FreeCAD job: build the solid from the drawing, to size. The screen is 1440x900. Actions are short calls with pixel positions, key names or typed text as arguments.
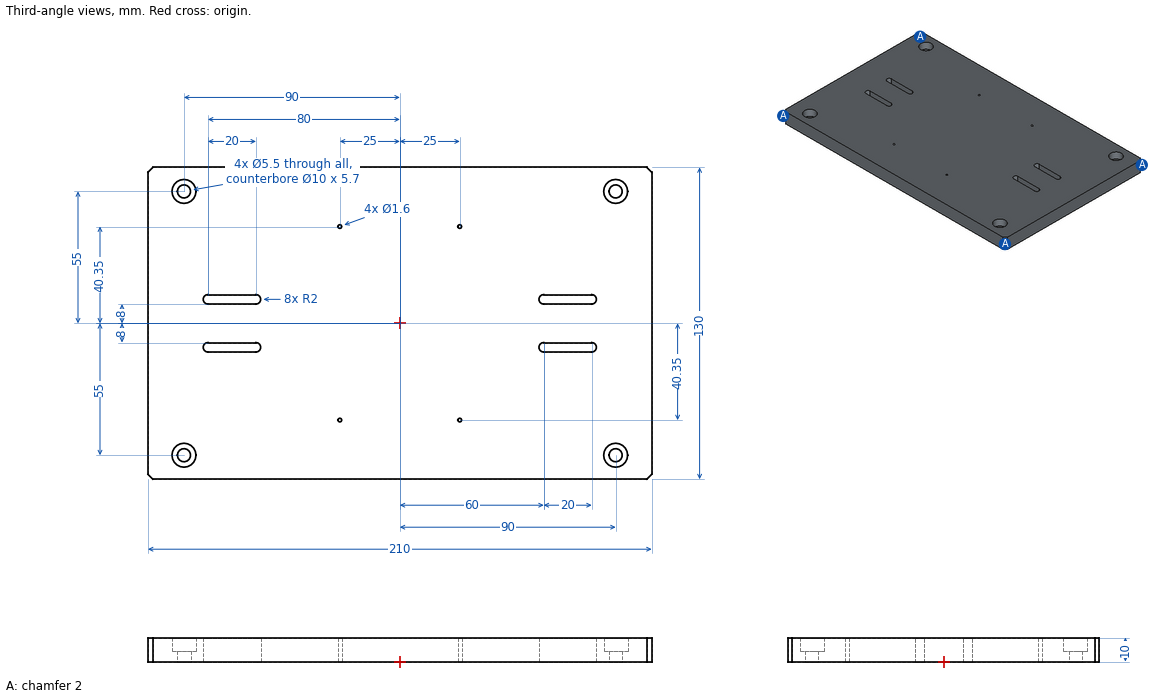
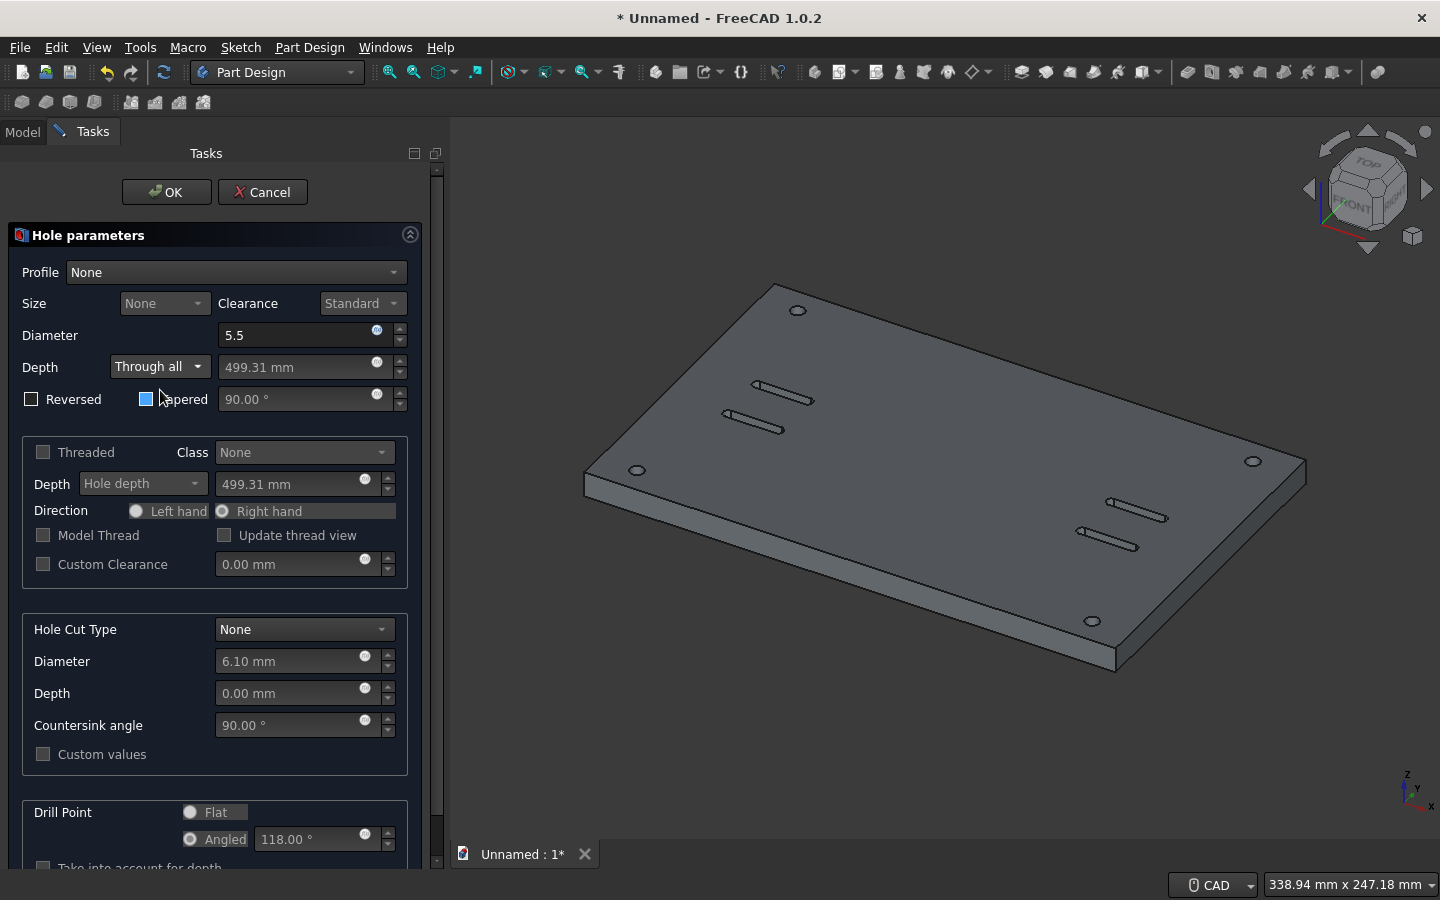
click(306, 630)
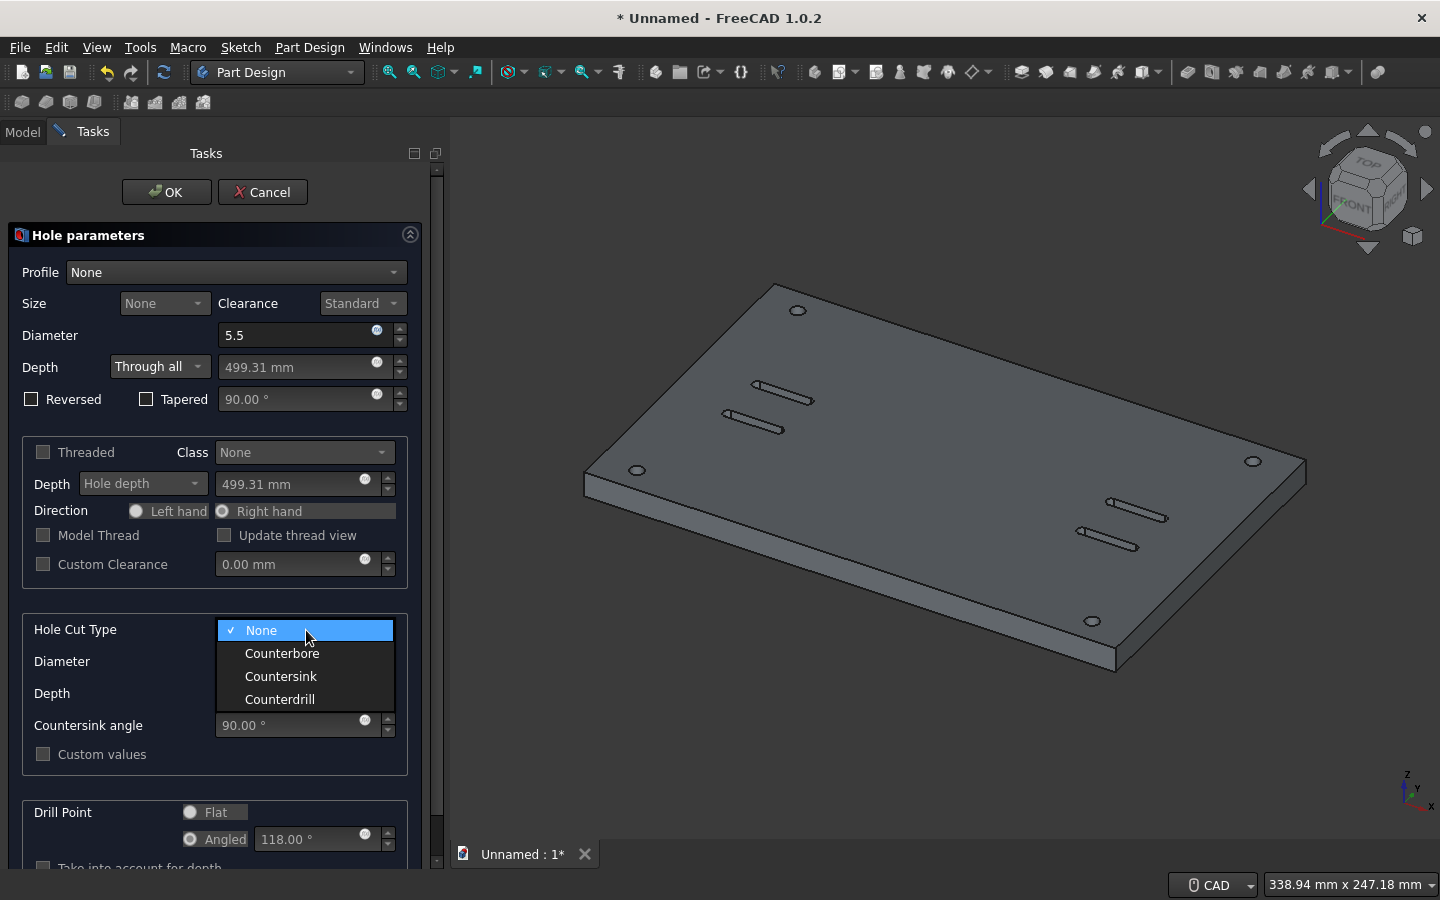
click(304, 654)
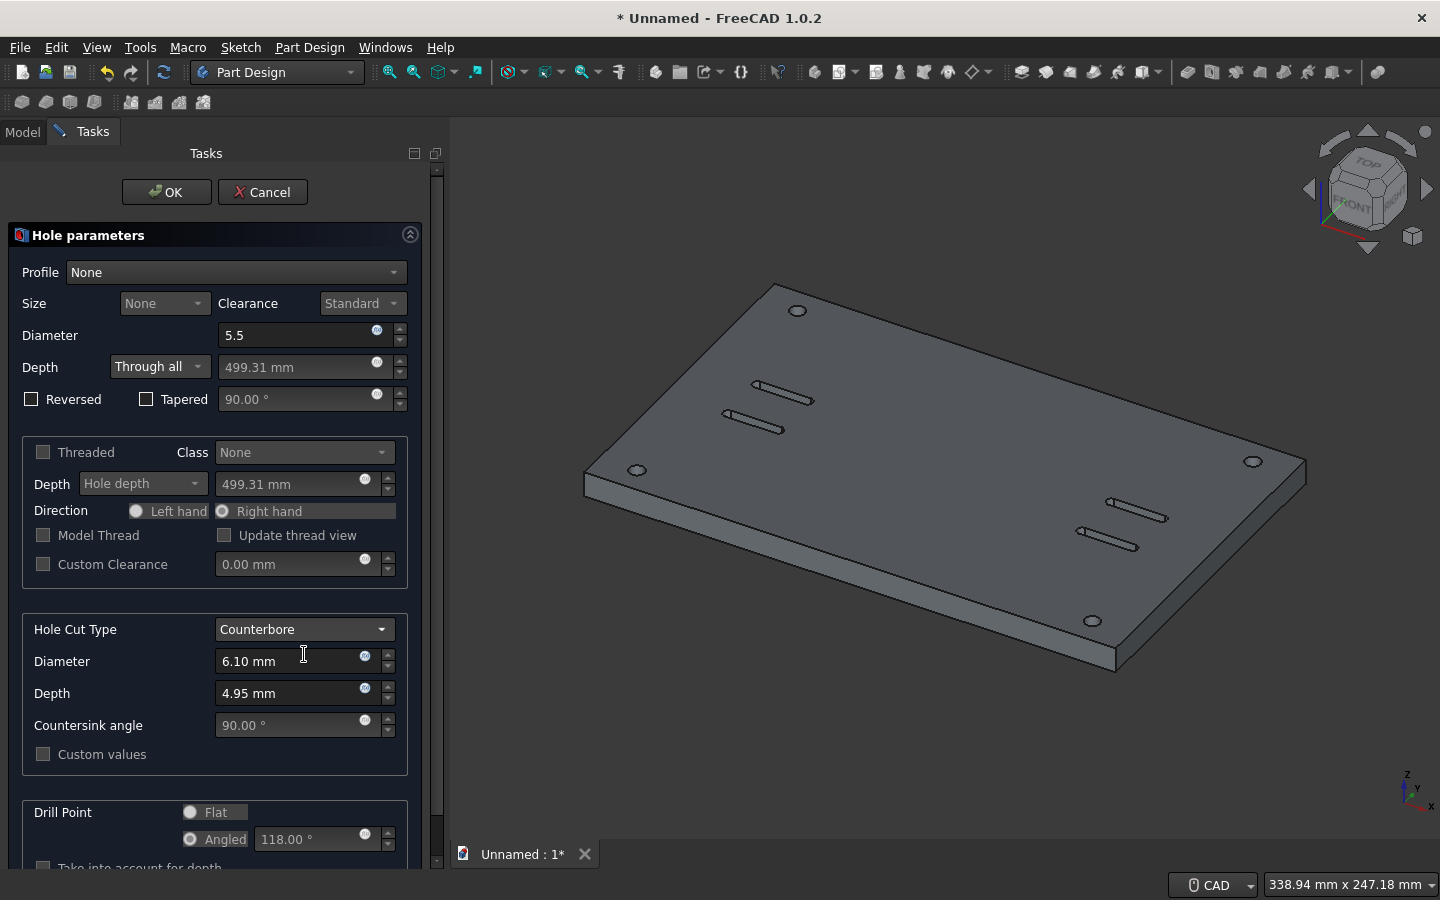
triple_click(298, 661)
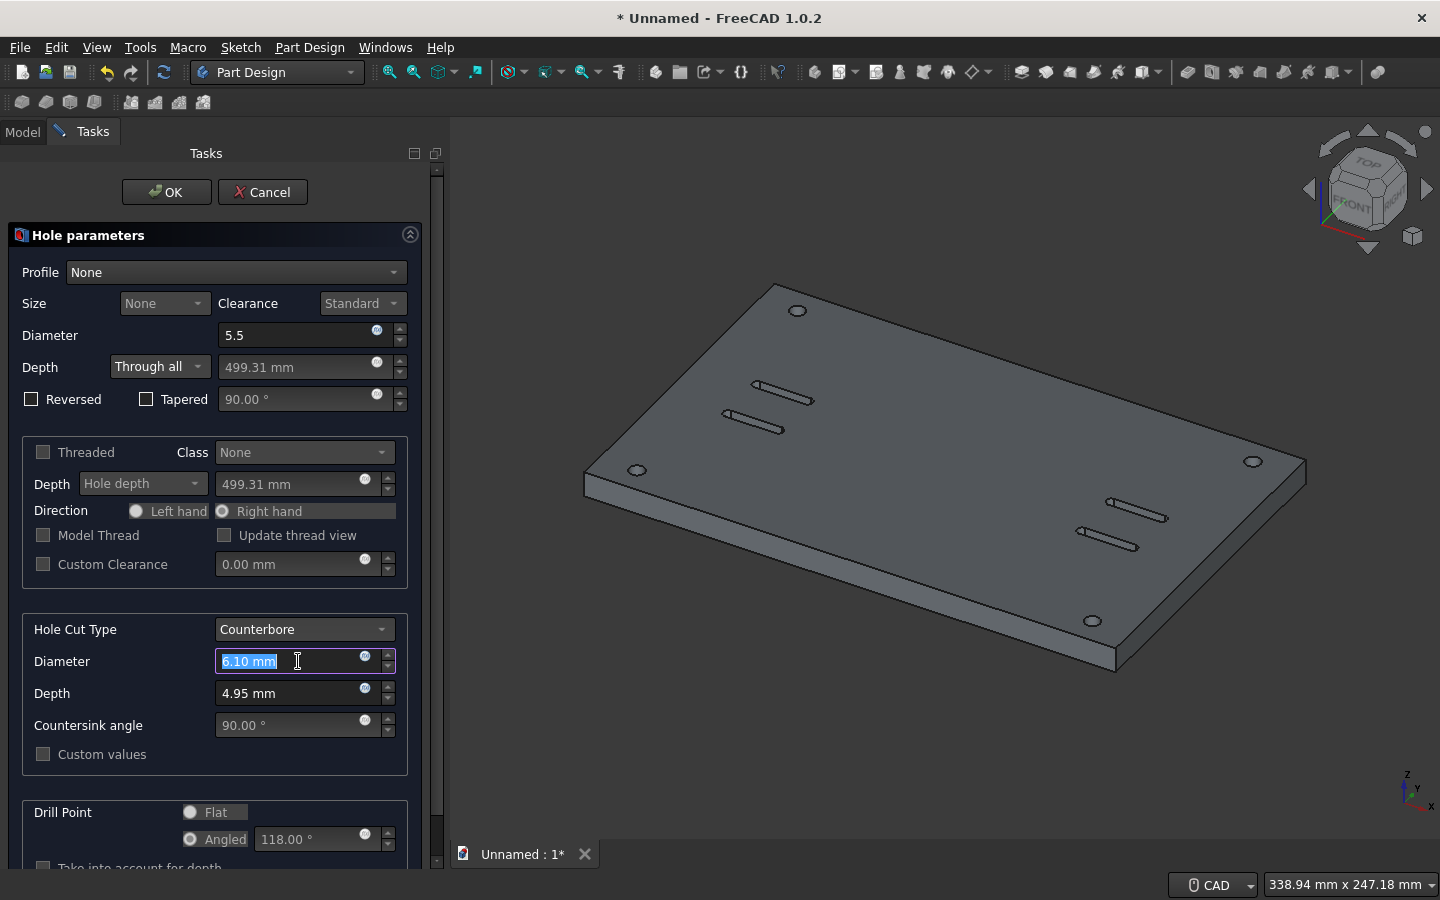
text(10)
key(Tab)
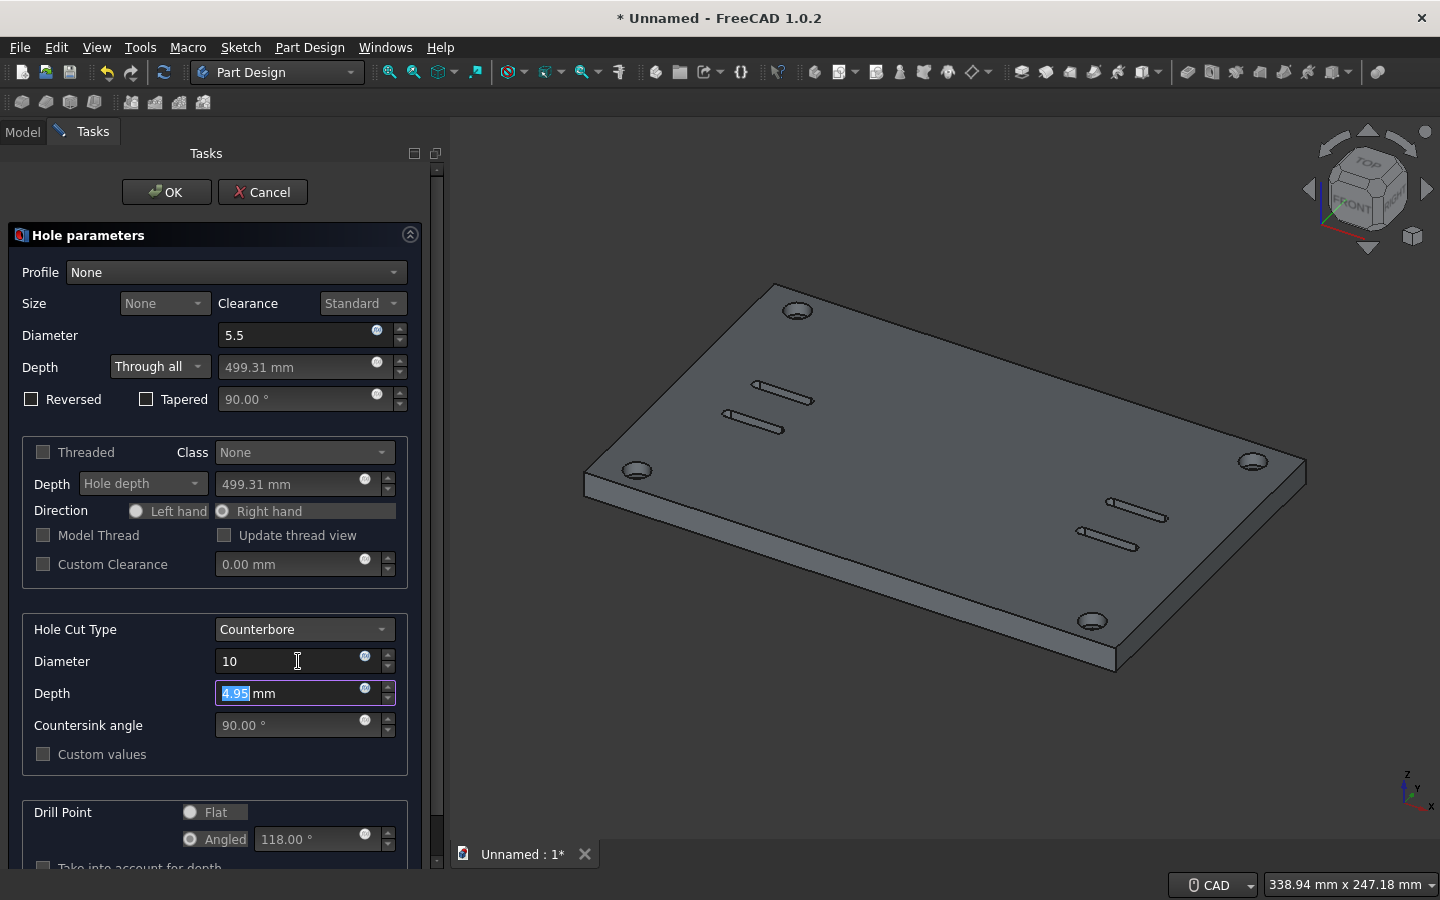
text(5.7)
key(Tab)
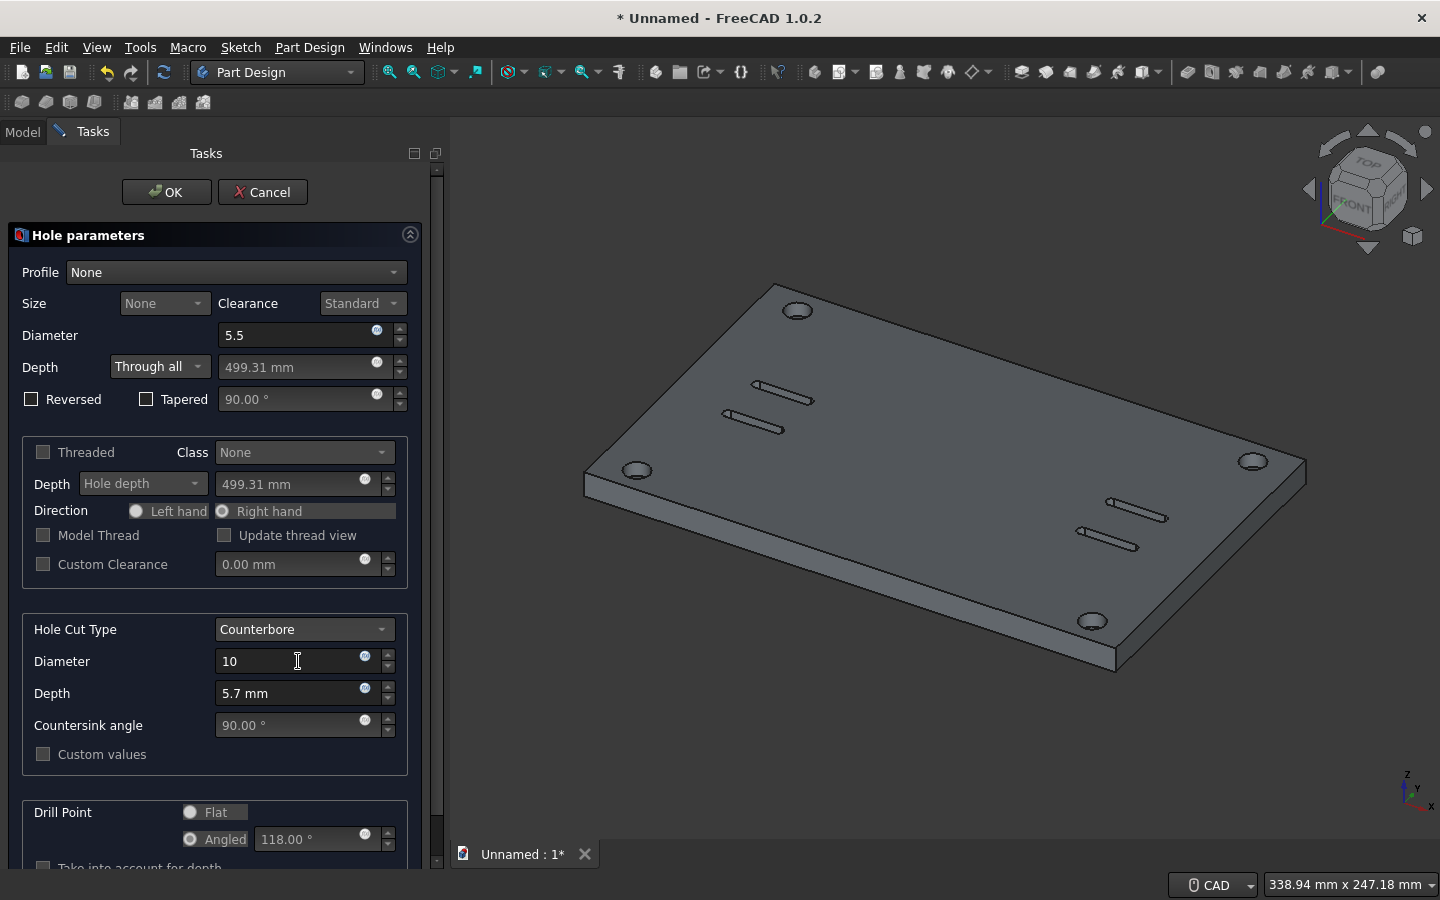
click(167, 192)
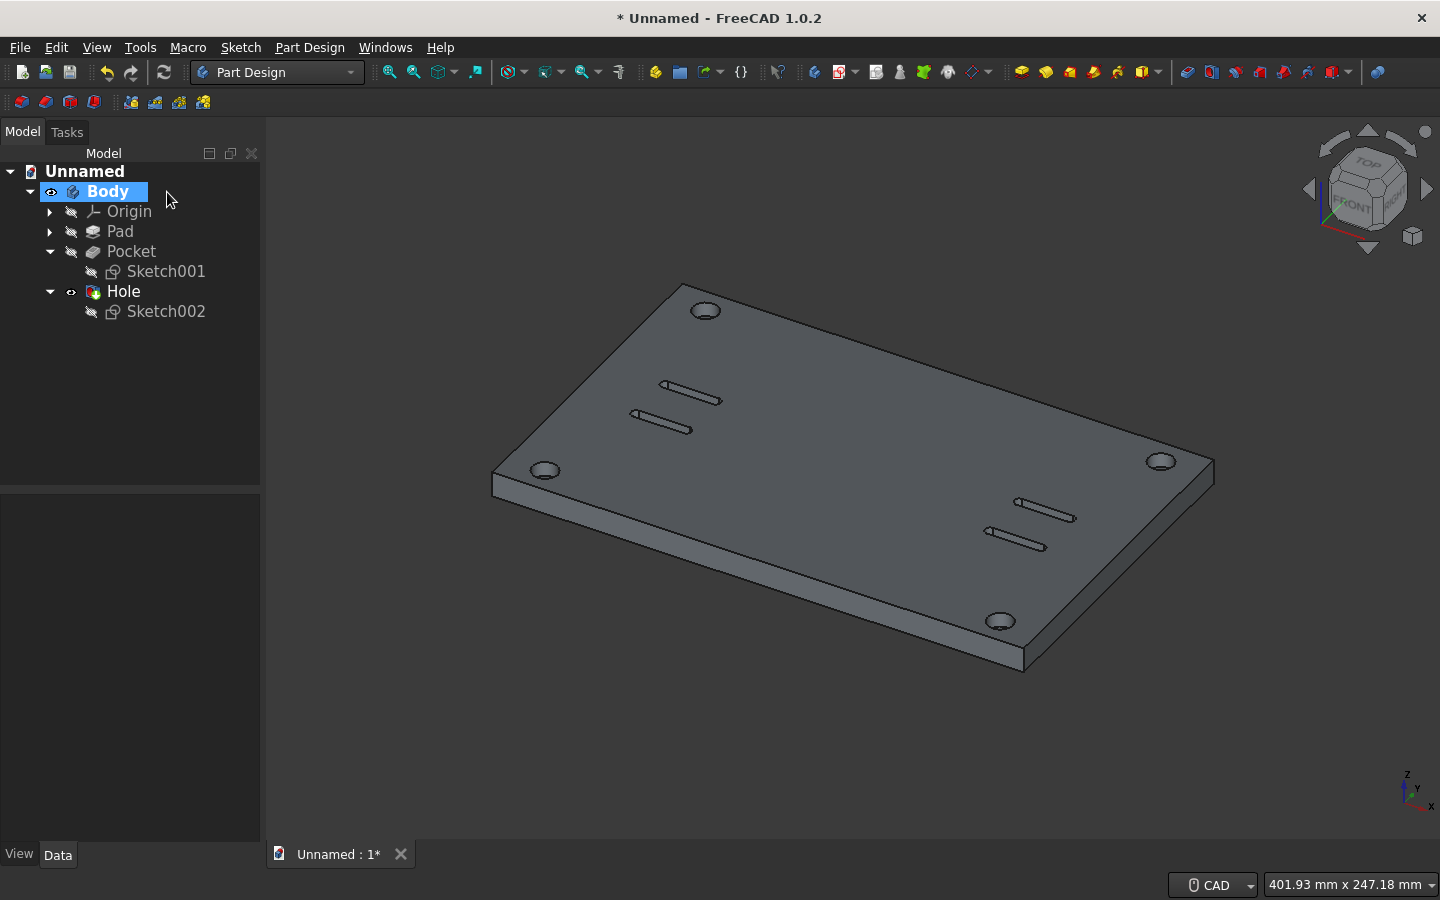
click(853, 465)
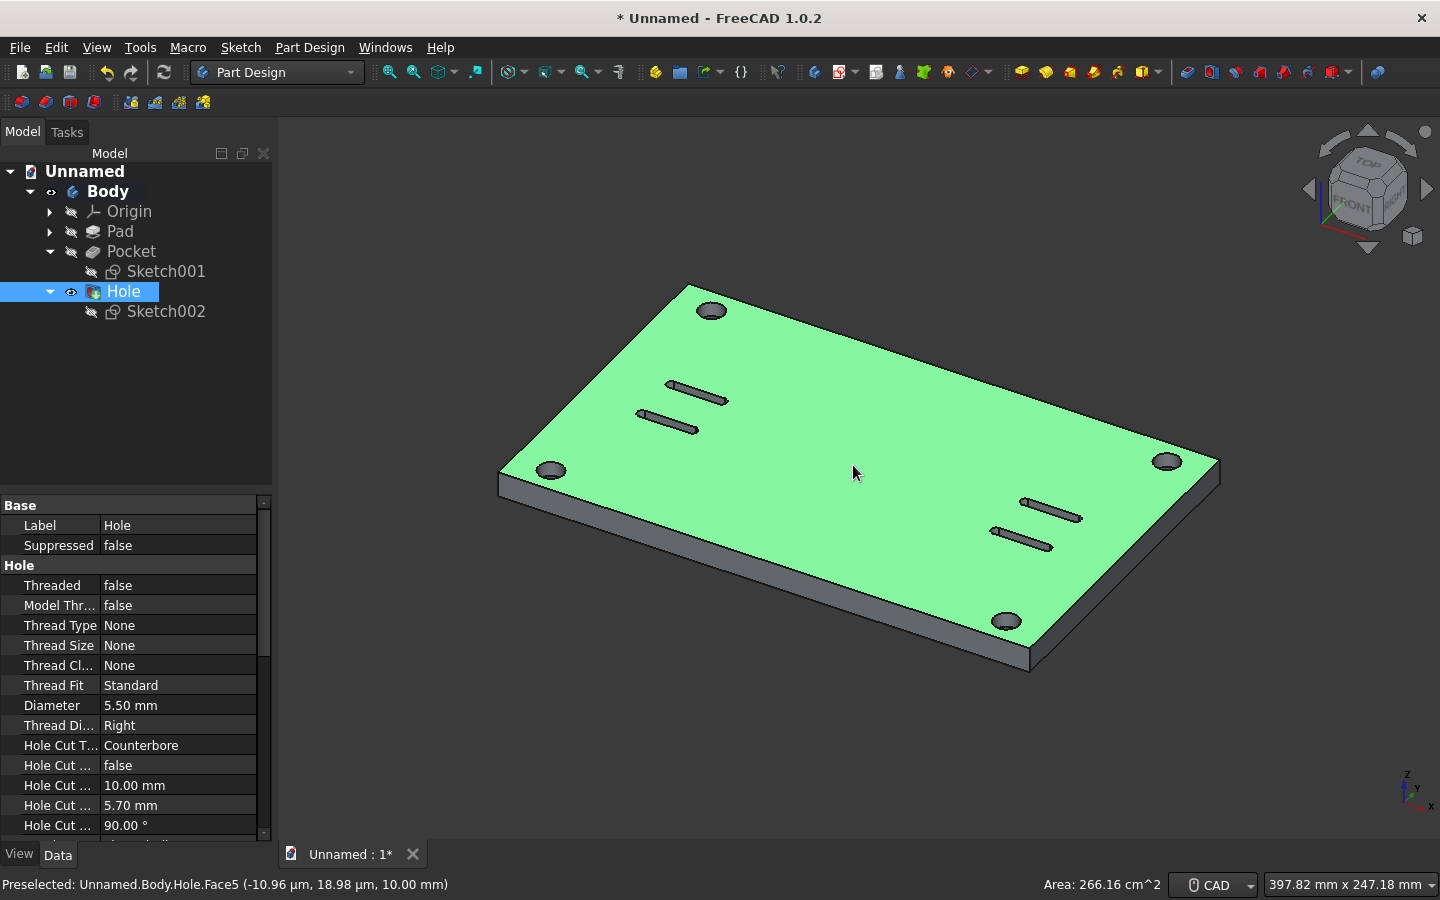
click(840, 72)